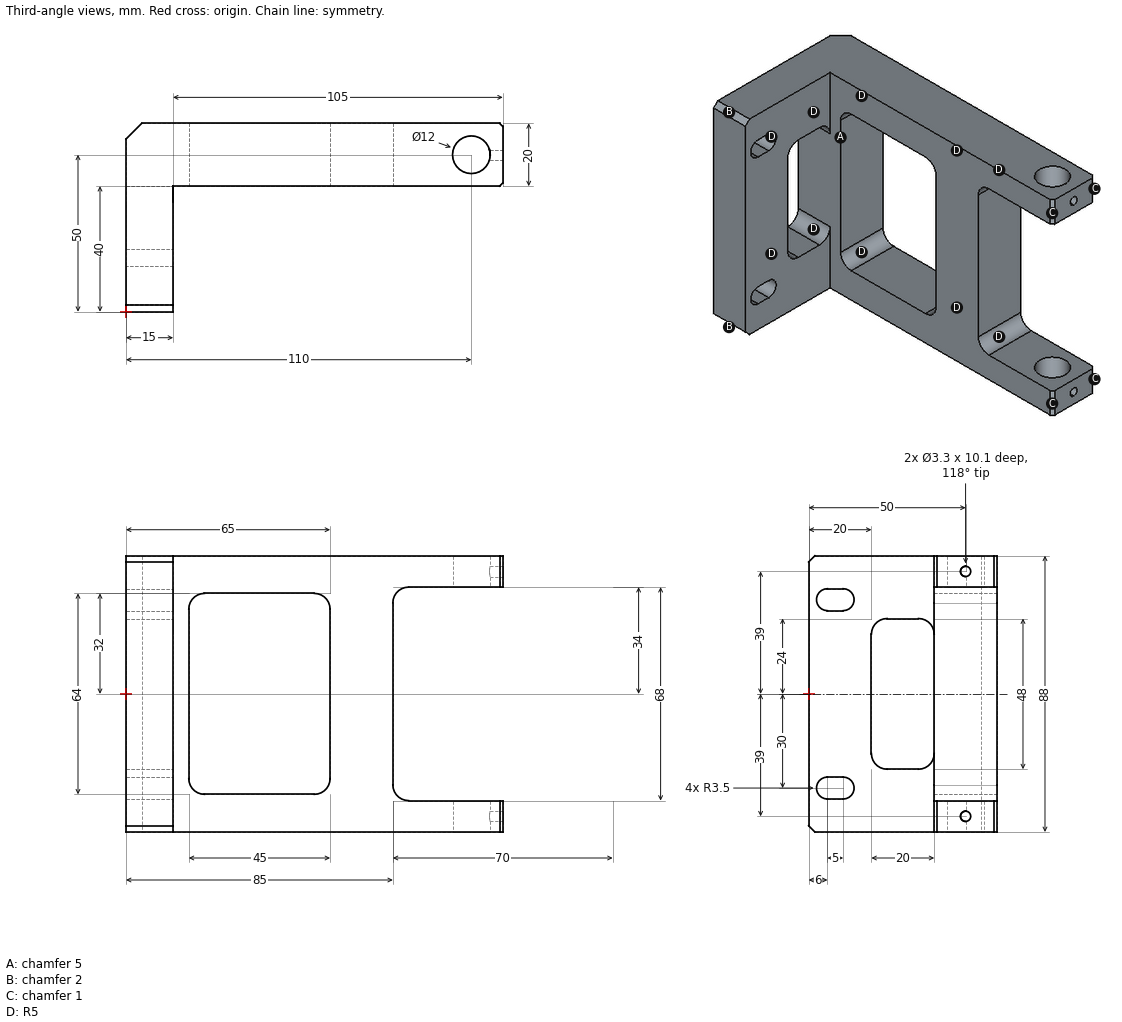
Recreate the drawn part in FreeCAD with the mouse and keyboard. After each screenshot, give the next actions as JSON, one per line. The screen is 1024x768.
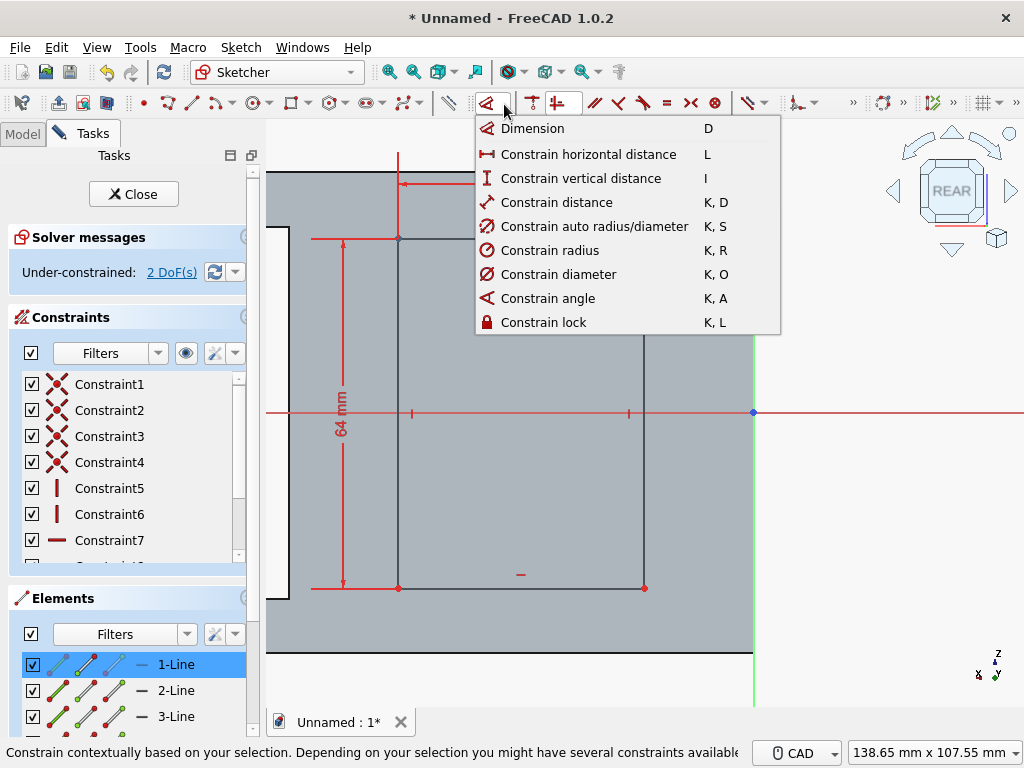
{"action": "left_click", "coordinate": [628, 154]}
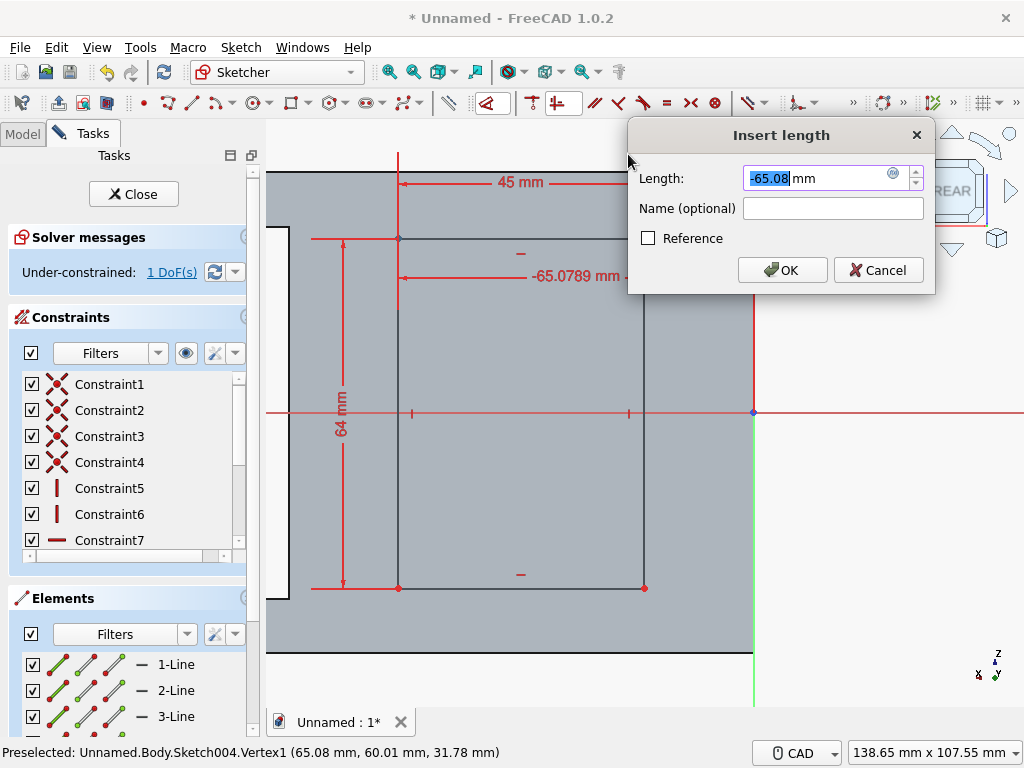
{"action": "type", "text": "-65"}
{"action": "key", "text": "Return"}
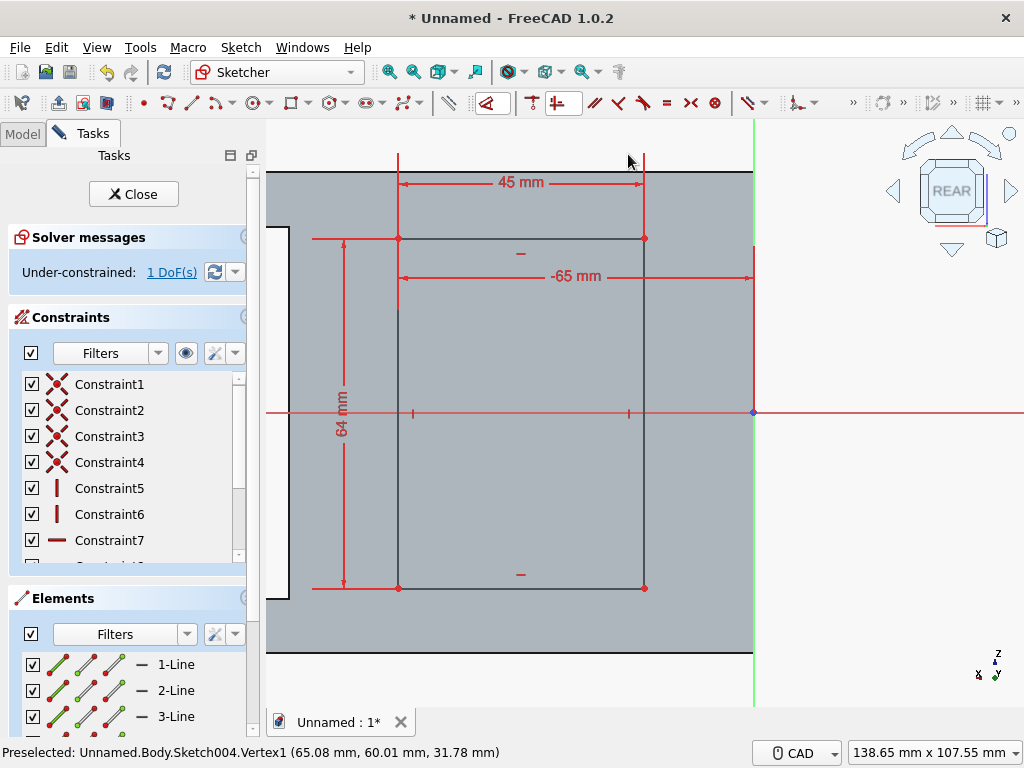
{"action": "left_click", "coordinate": [398, 239]}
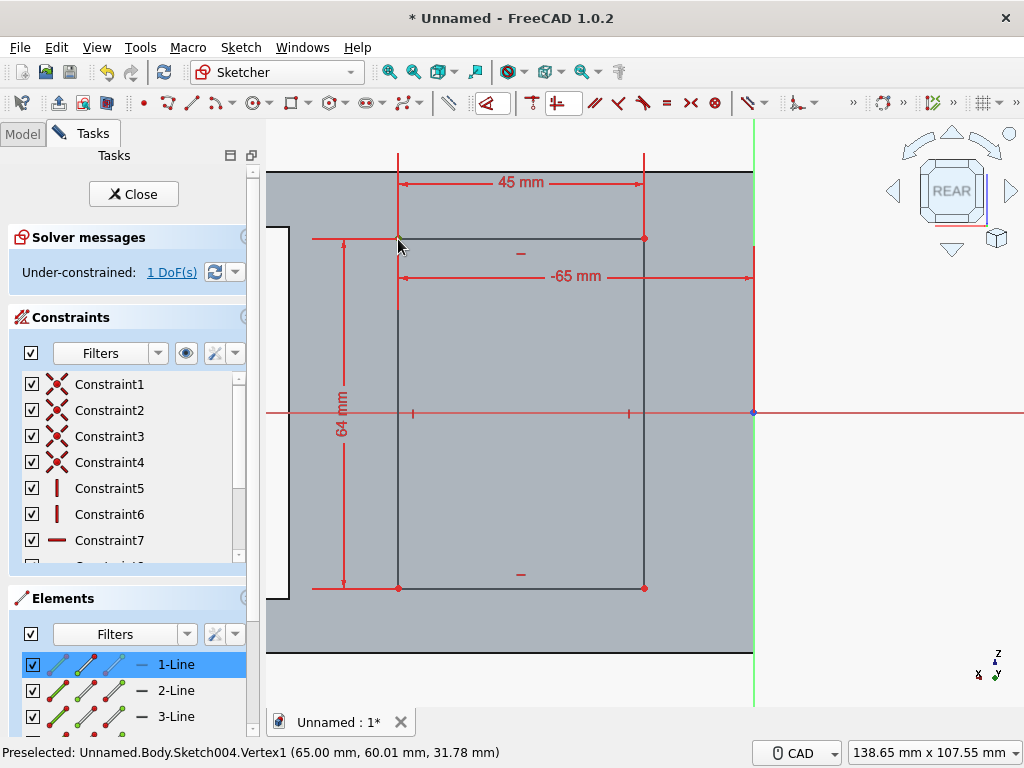
{"action": "left_click", "coordinate": [504, 104]}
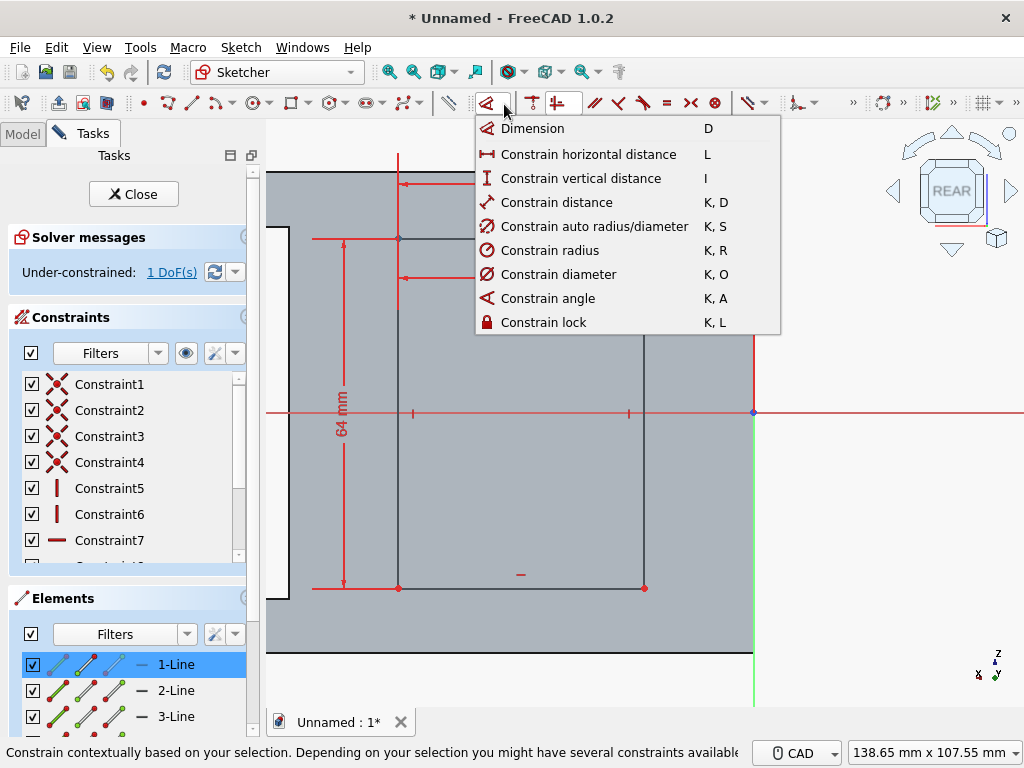
{"action": "left_click", "coordinate": [628, 178]}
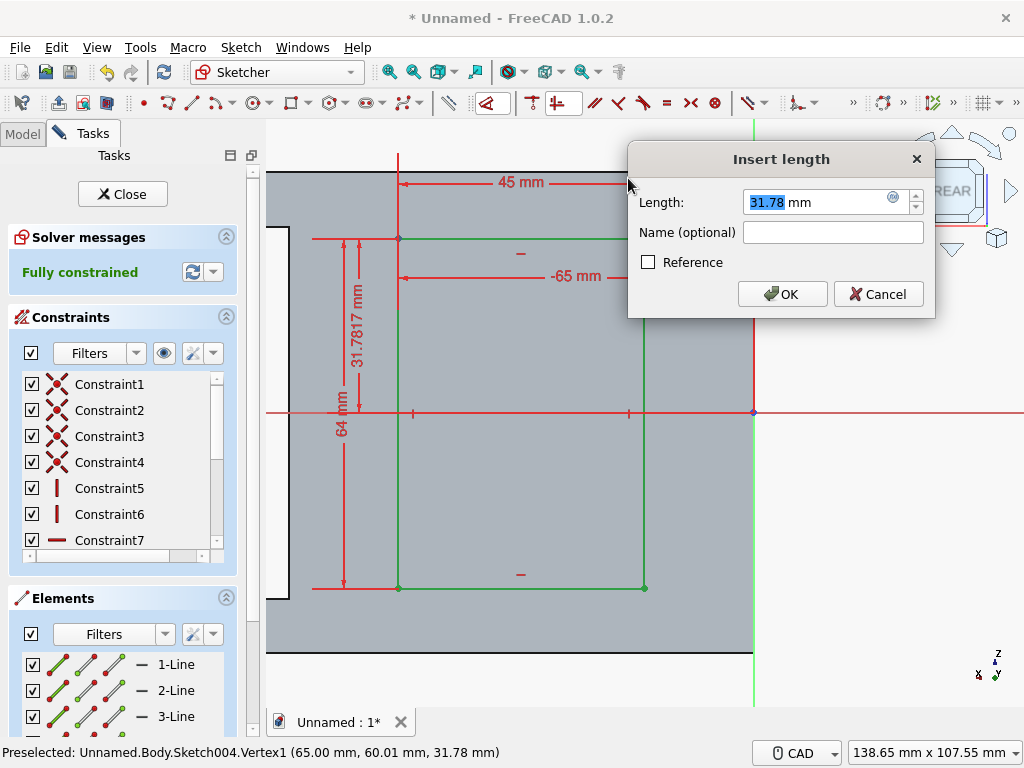
{"action": "type", "text": "32"}
{"action": "key", "text": "Return"}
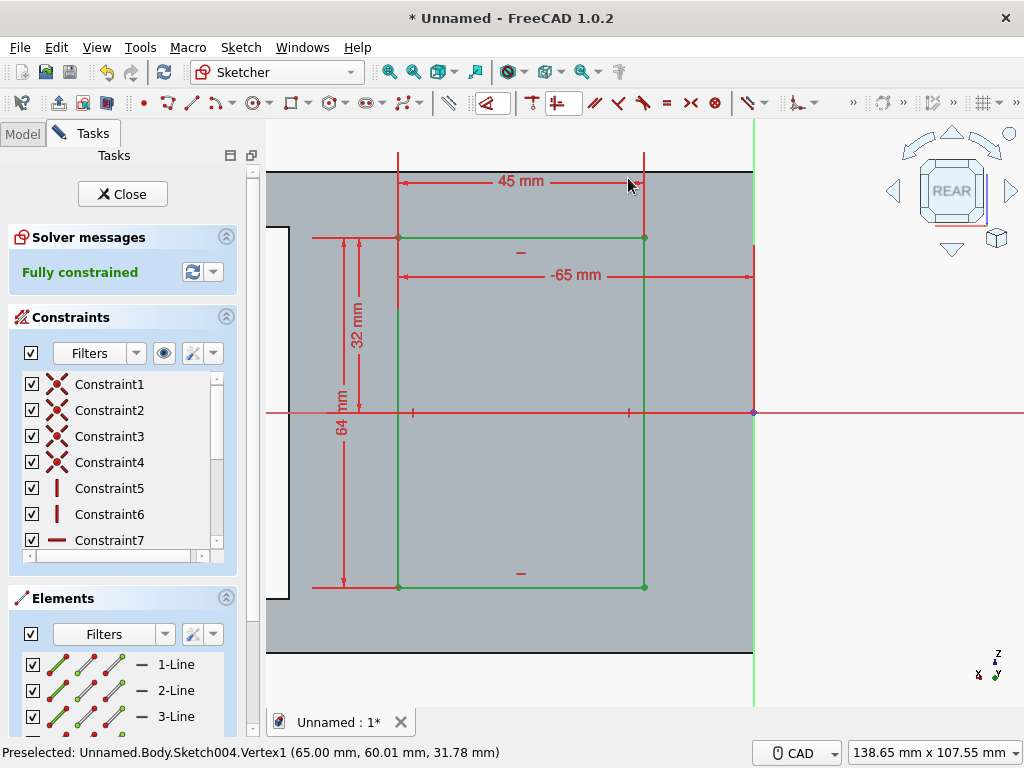
{"action": "left_click", "coordinate": [123, 194]}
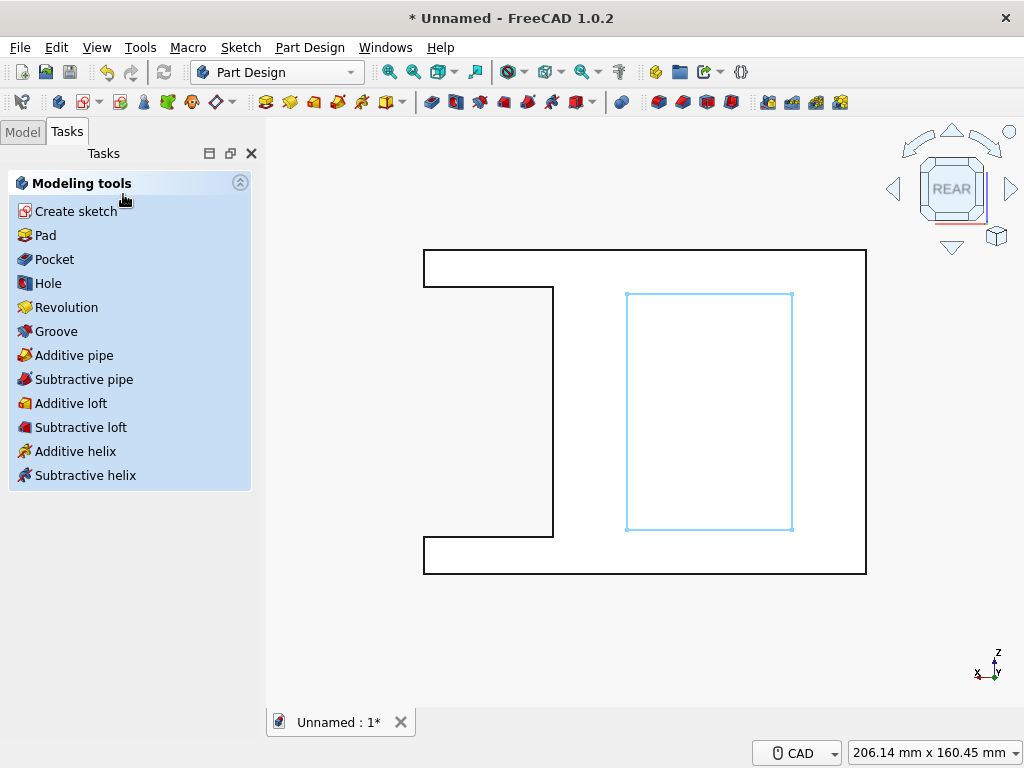
{"action": "left_click", "coordinate": [432, 102]}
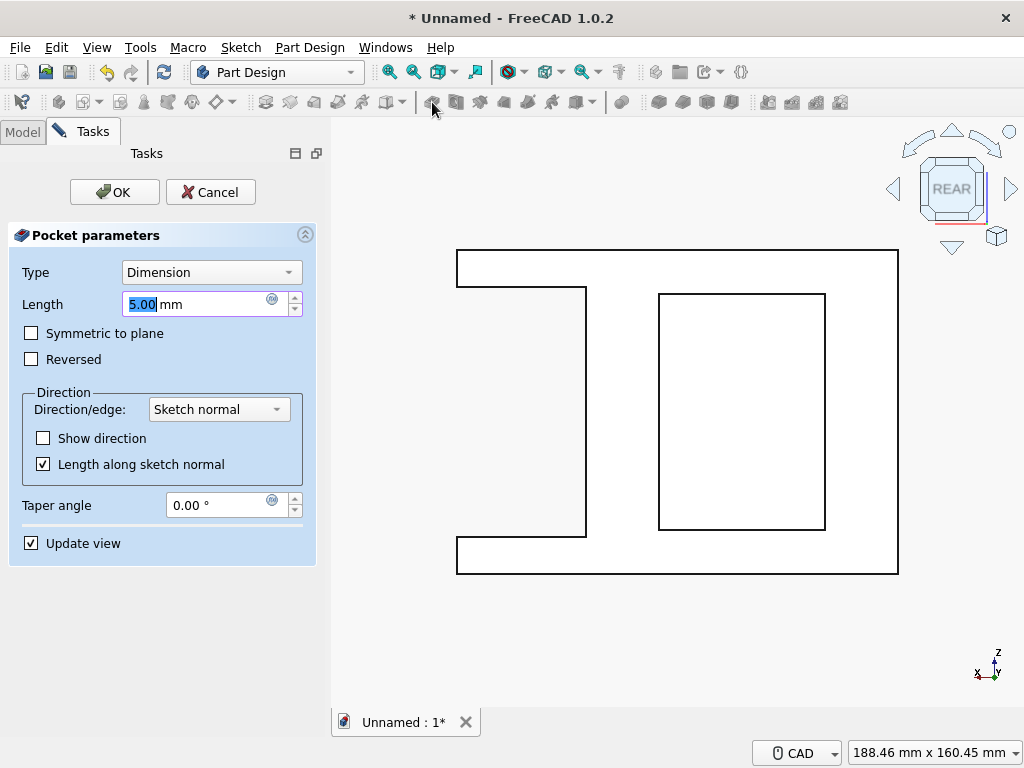
{"action": "left_click", "coordinate": [212, 272]}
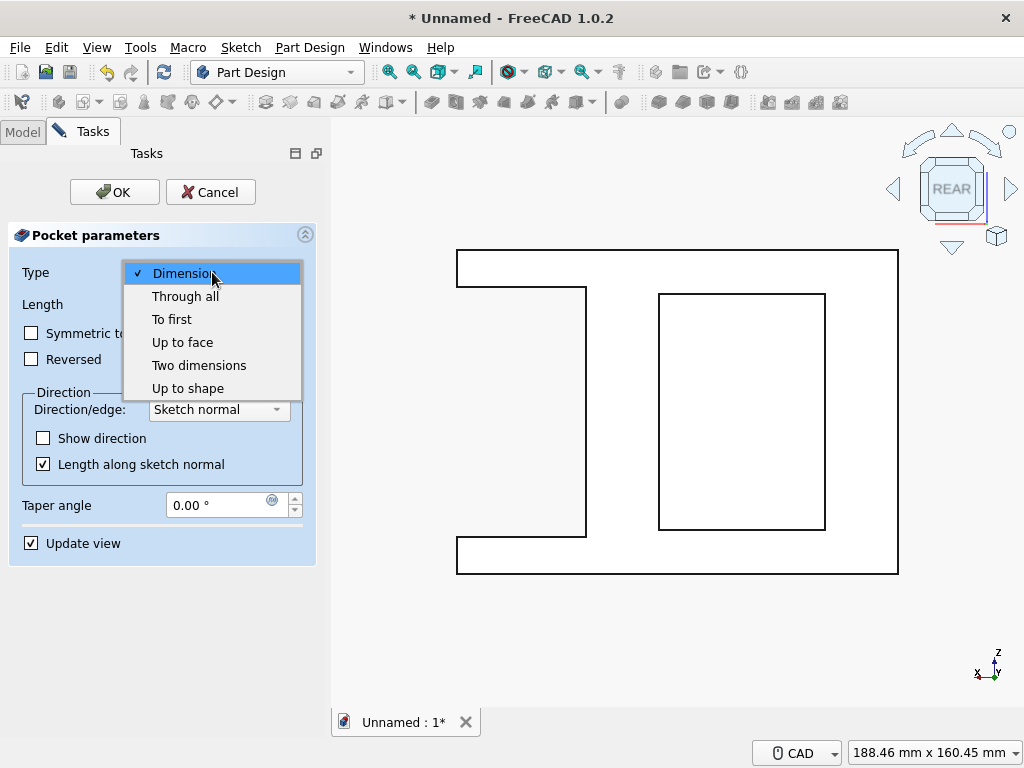
{"action": "left_click", "coordinate": [212, 296]}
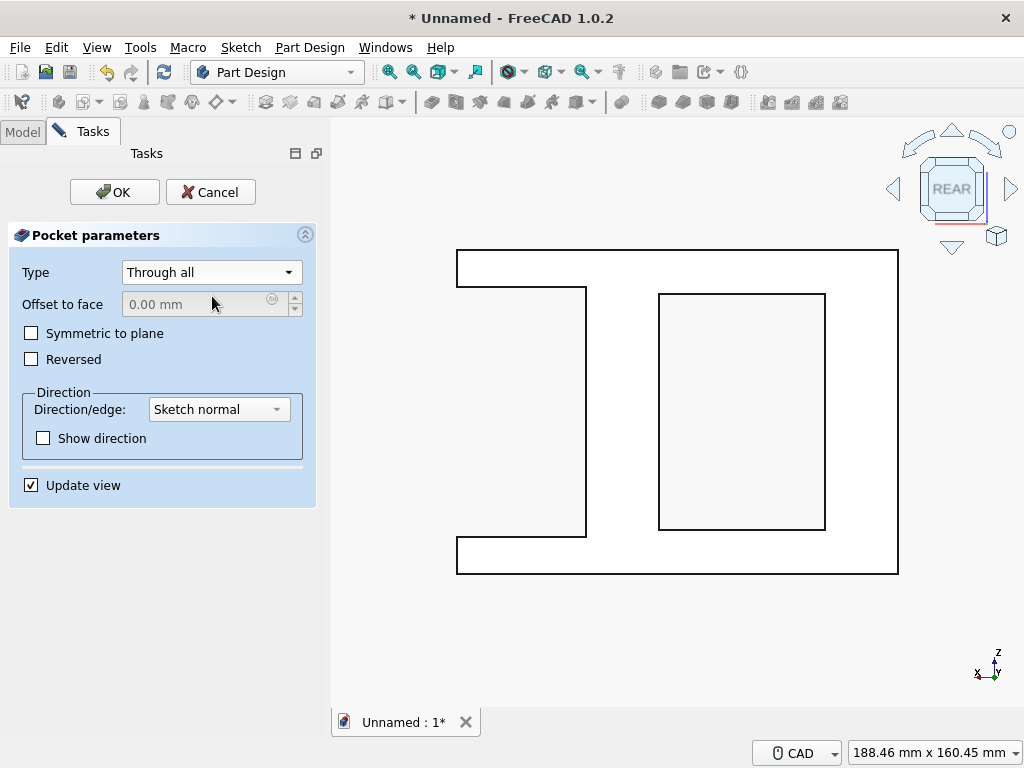
{"action": "left_click", "coordinate": [115, 192]}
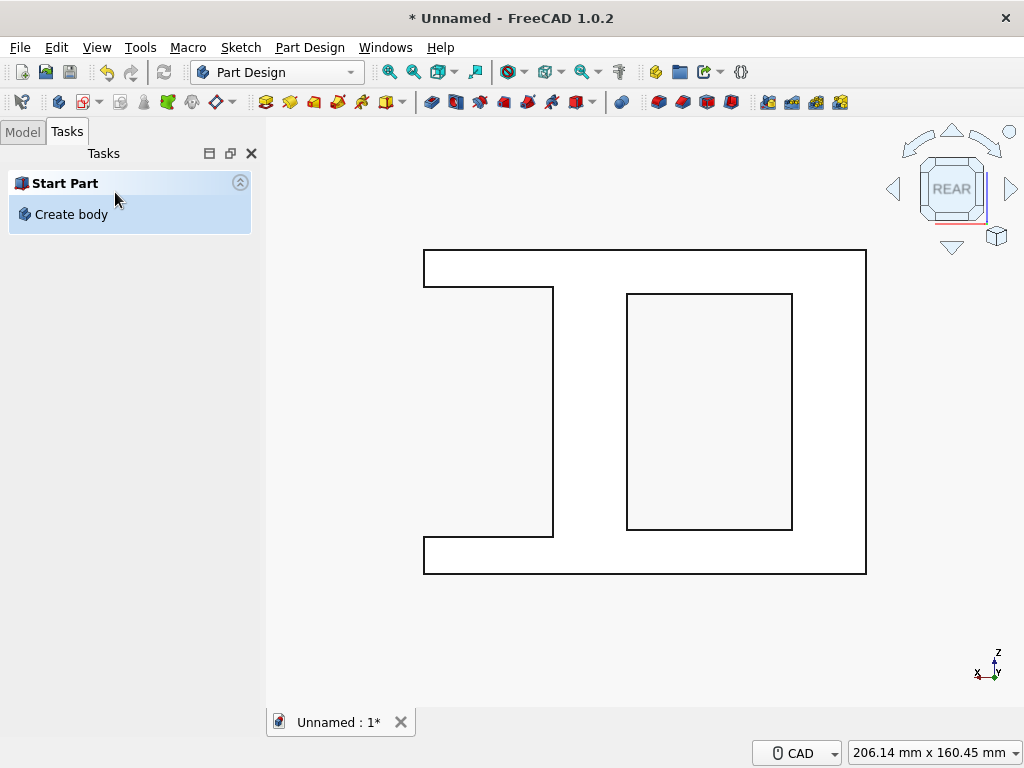
{"action": "left_click", "coordinate": [84, 102]}